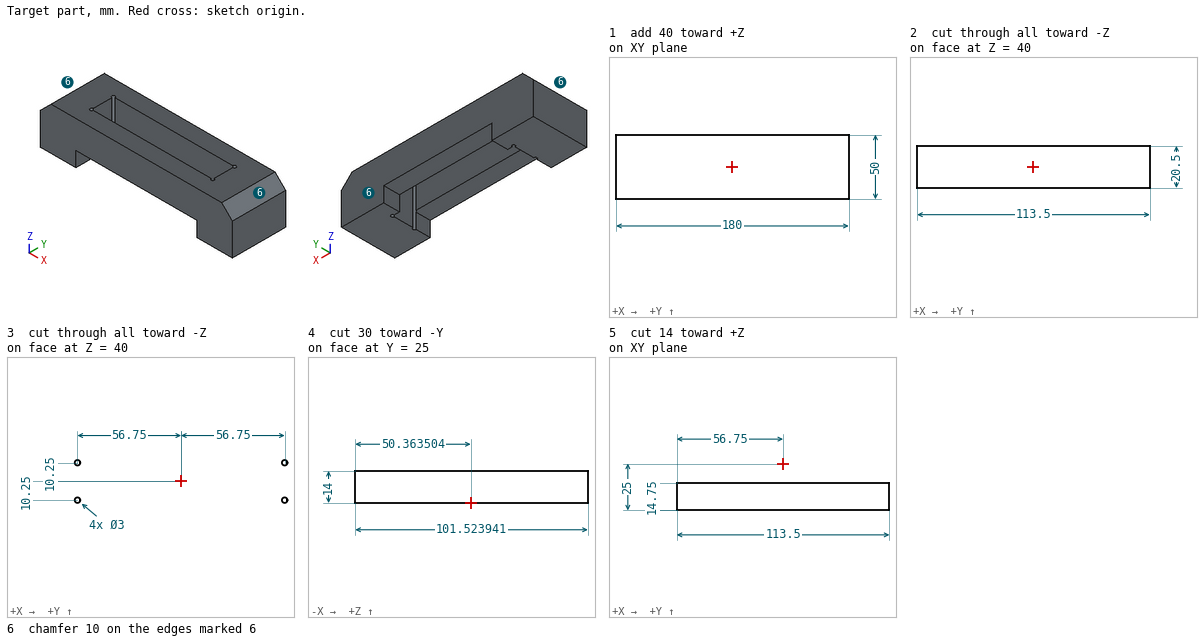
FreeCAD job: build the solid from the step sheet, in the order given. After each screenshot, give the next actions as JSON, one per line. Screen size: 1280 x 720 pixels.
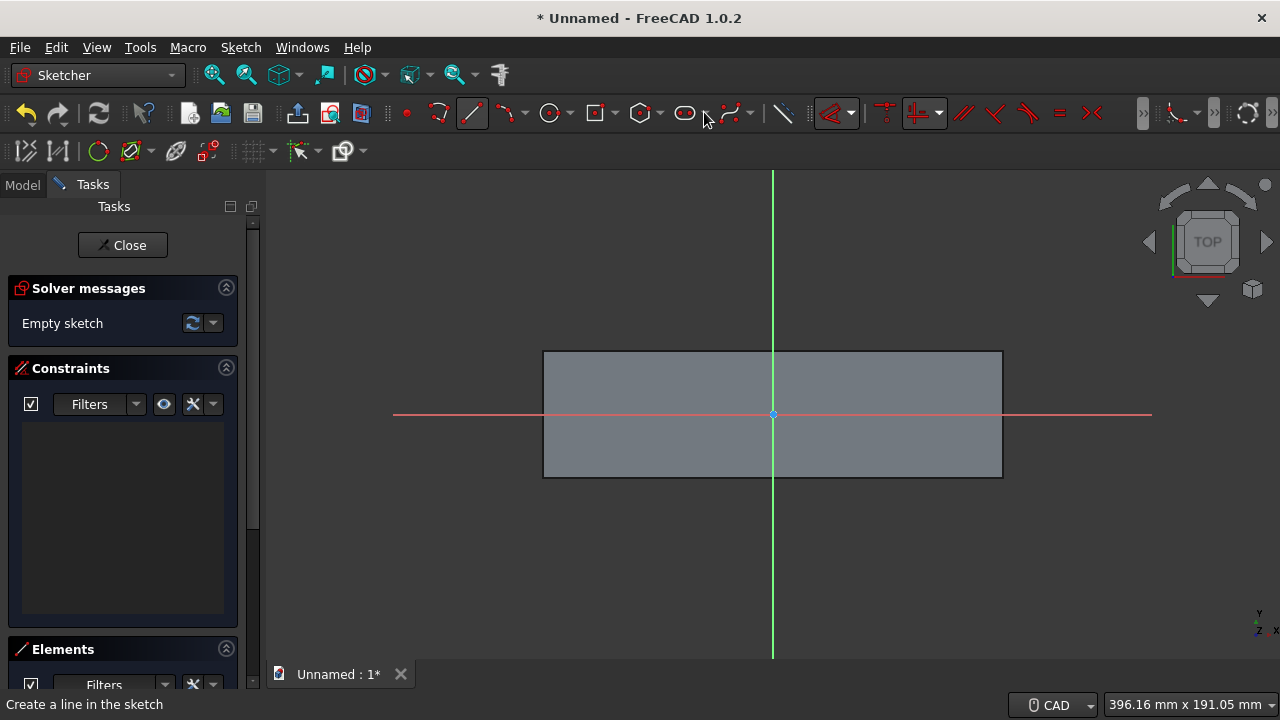
{"action": "scroll", "coordinate": [856, 415], "scroll_direction": "up", "scroll_amount": 3}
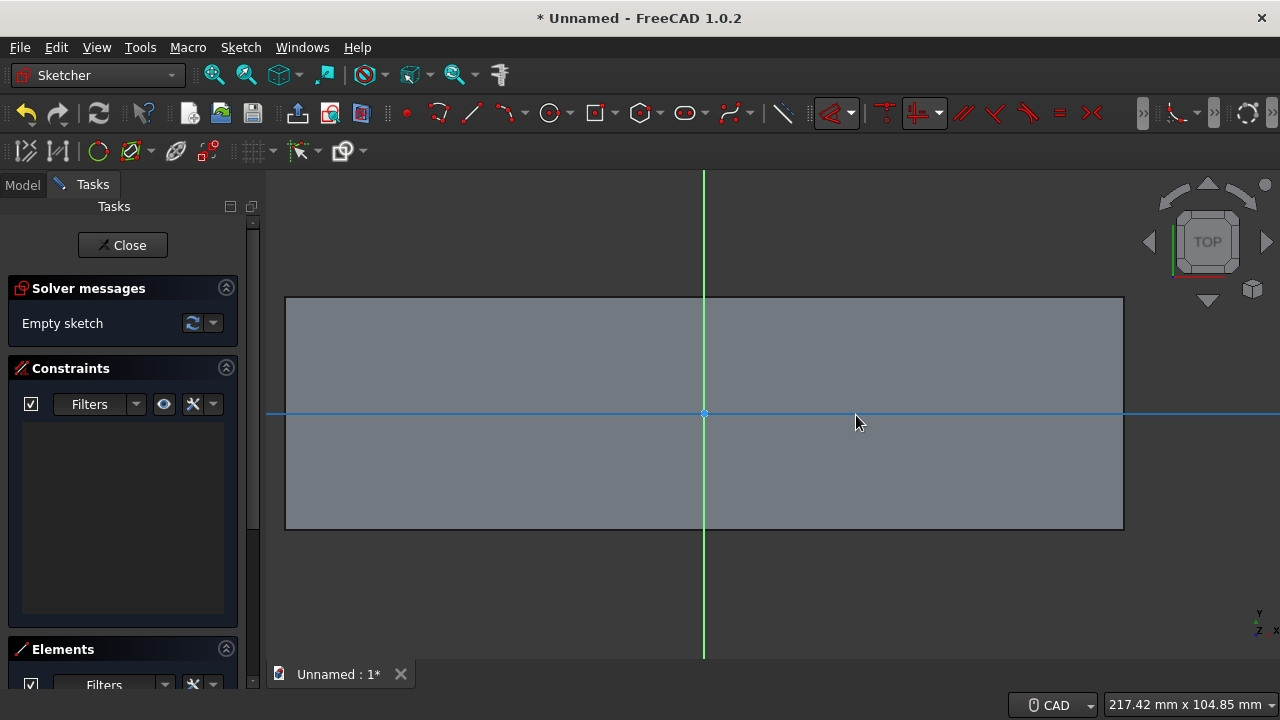
{"action": "key", "text": "g v"}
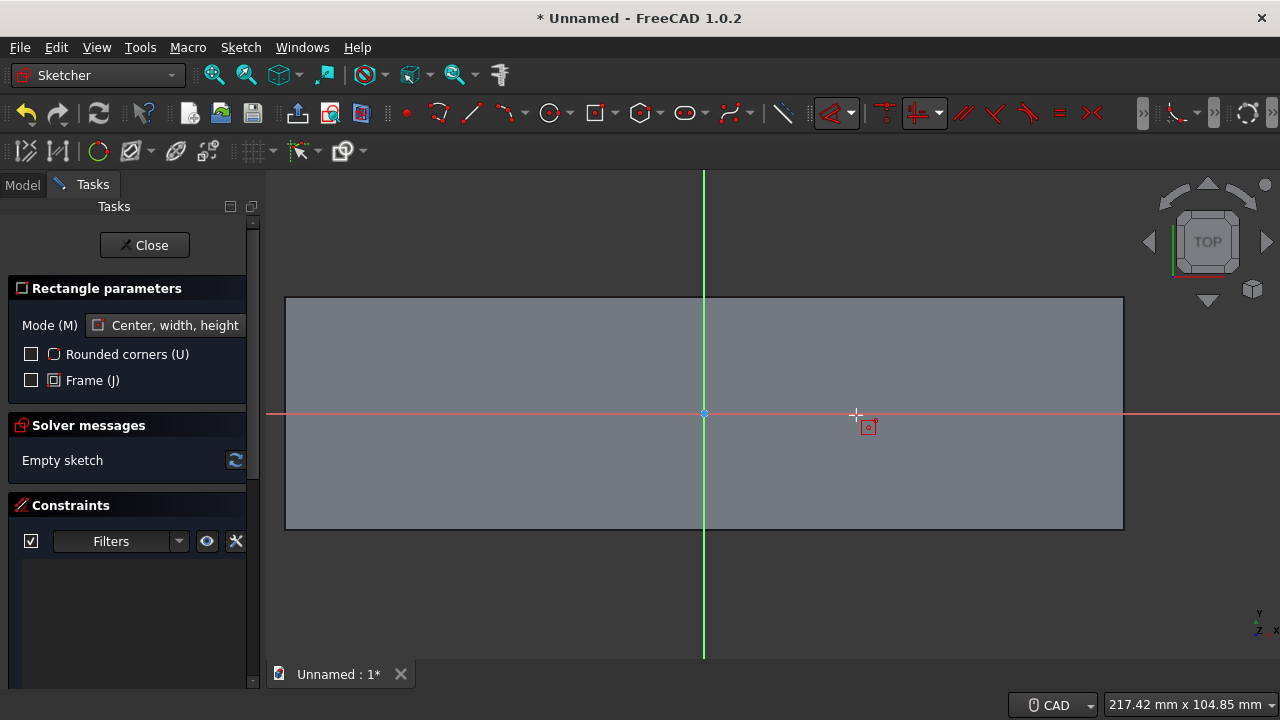
{"action": "left_click", "coordinate": [704, 414]}
{"action": "left_click", "coordinate": [969, 366]}
{"action": "key", "text": "Escape"}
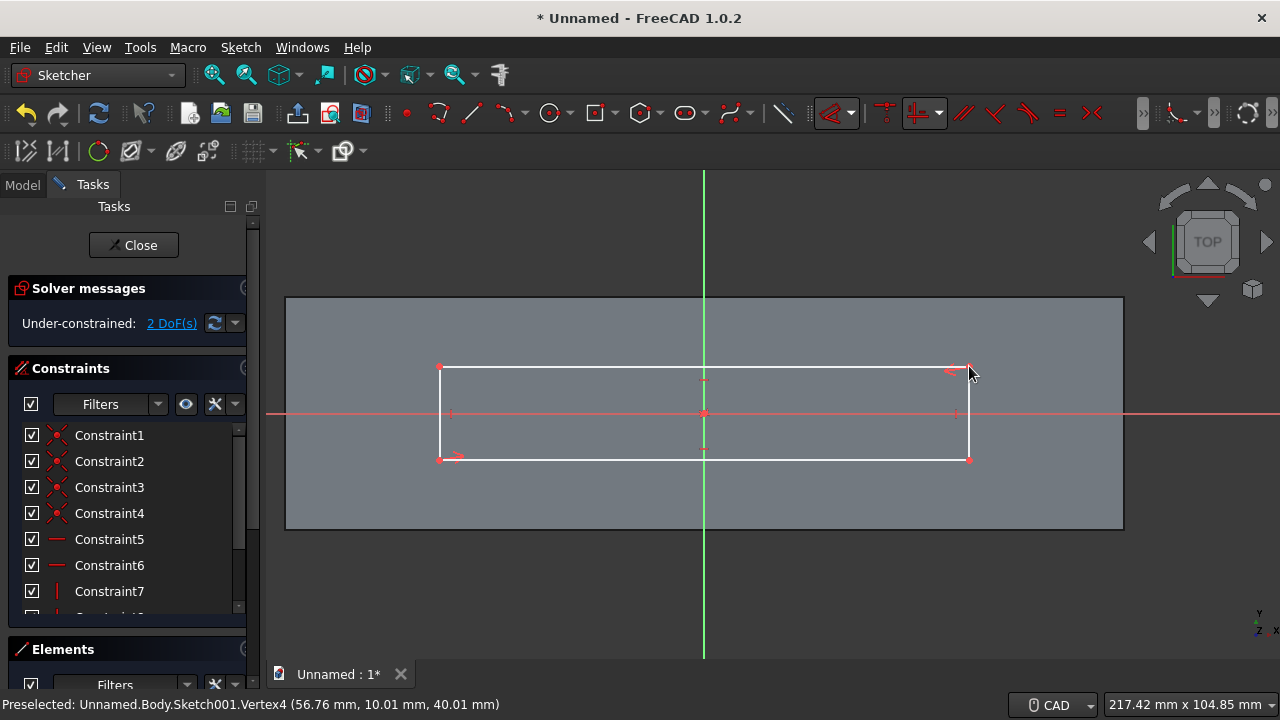
{"action": "left_click", "coordinate": [969, 432]}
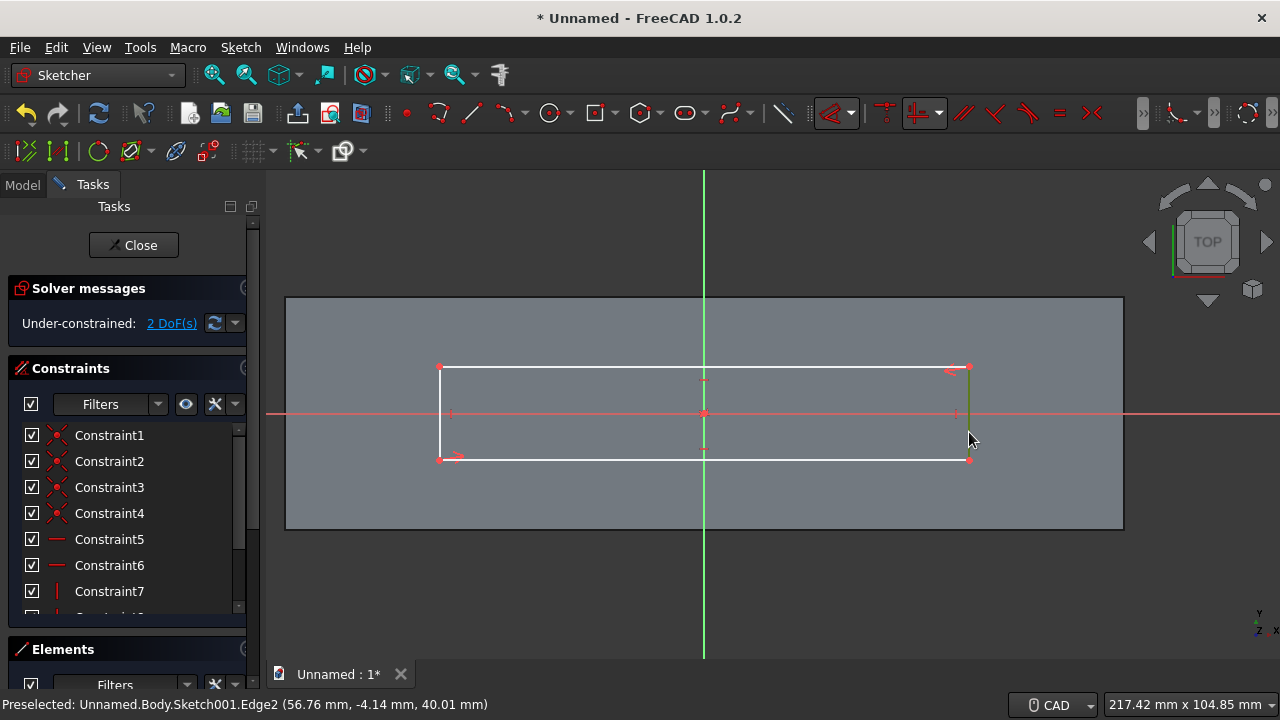
{"action": "key", "text": "i"}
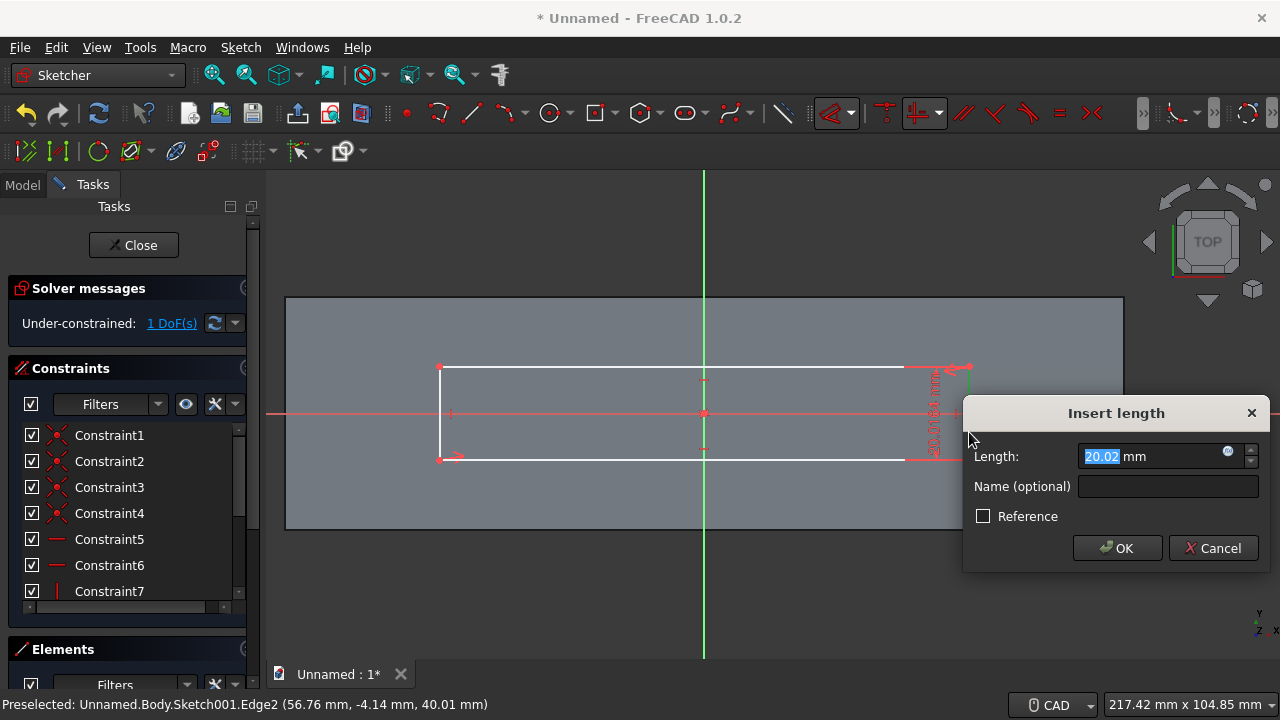
{"action": "type", "text": "20.5"}
{"action": "key", "text": "Return"}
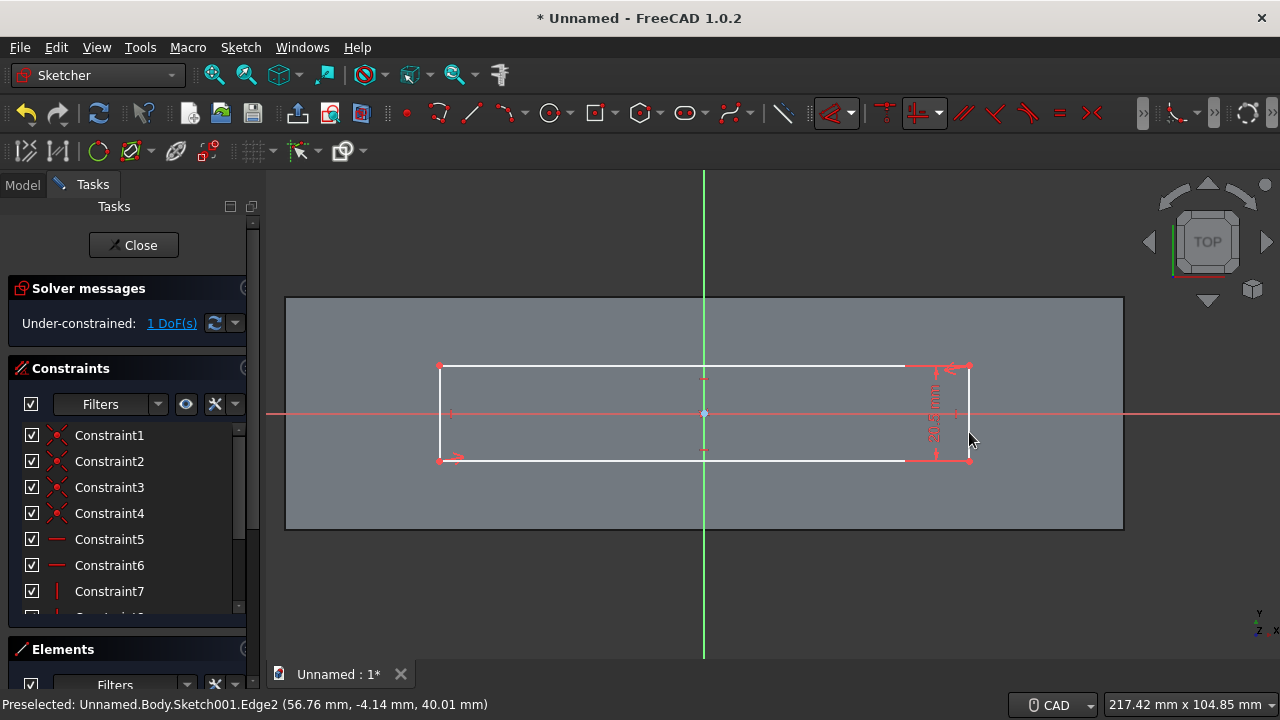
{"action": "left_click", "coordinate": [598, 461]}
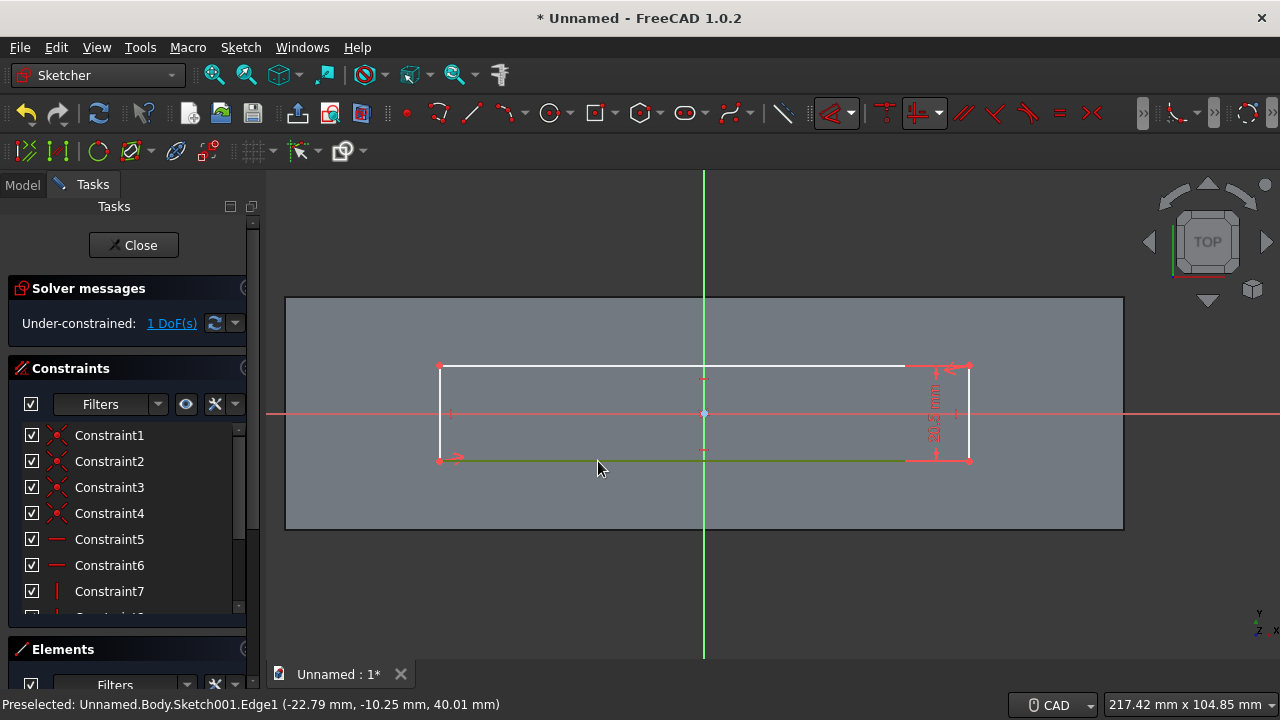
{"action": "left_click", "coordinate": [854, 114]}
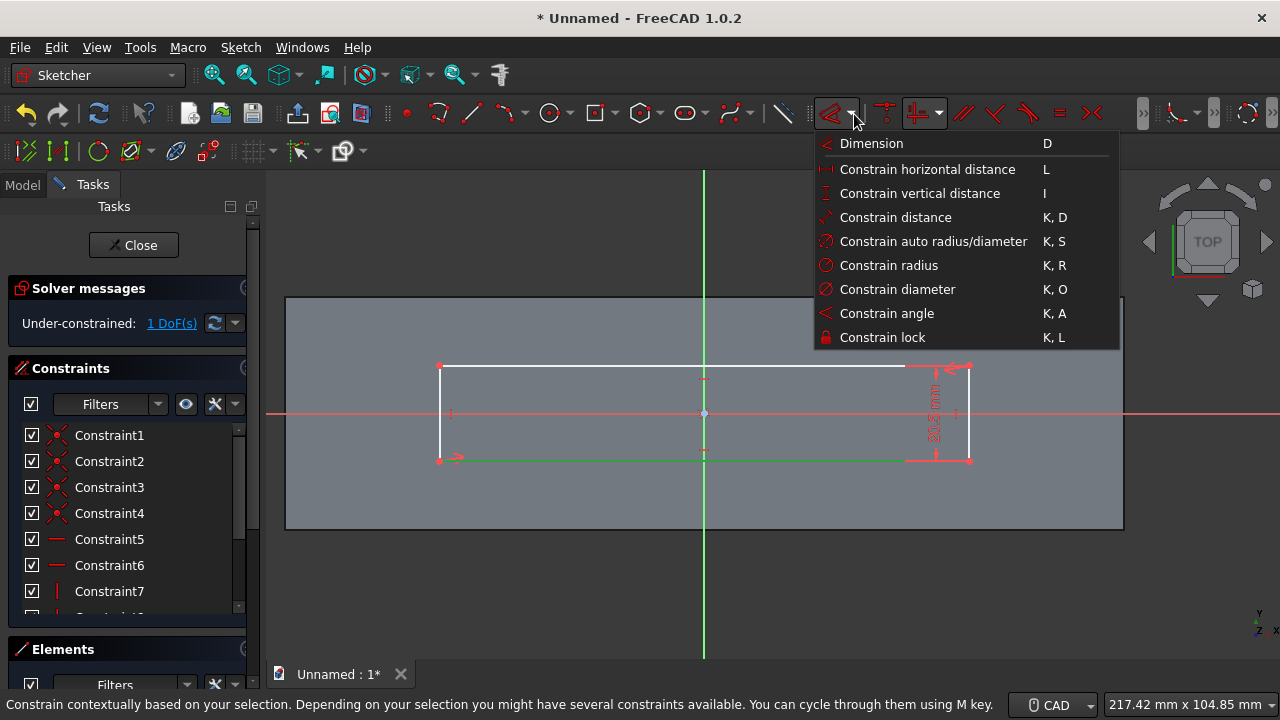
{"action": "left_click", "coordinate": [967, 169]}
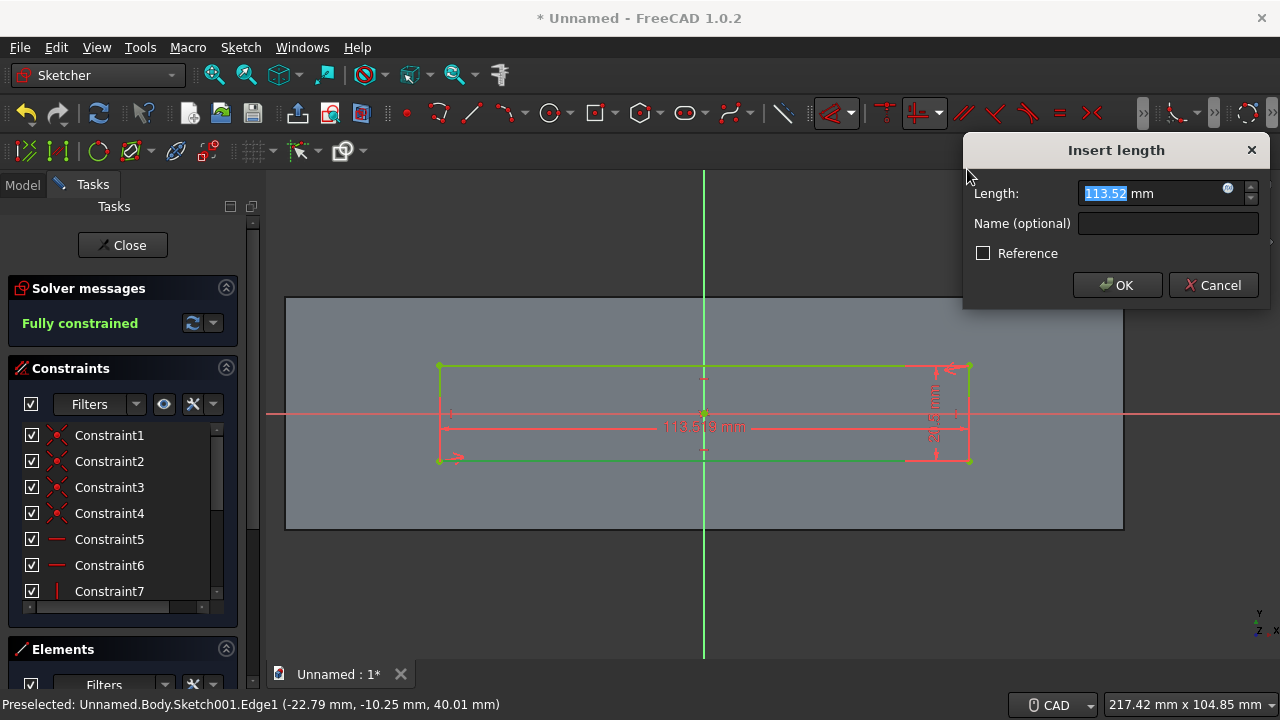
{"action": "type", "text": "113.5"}
{"action": "key", "text": "Return"}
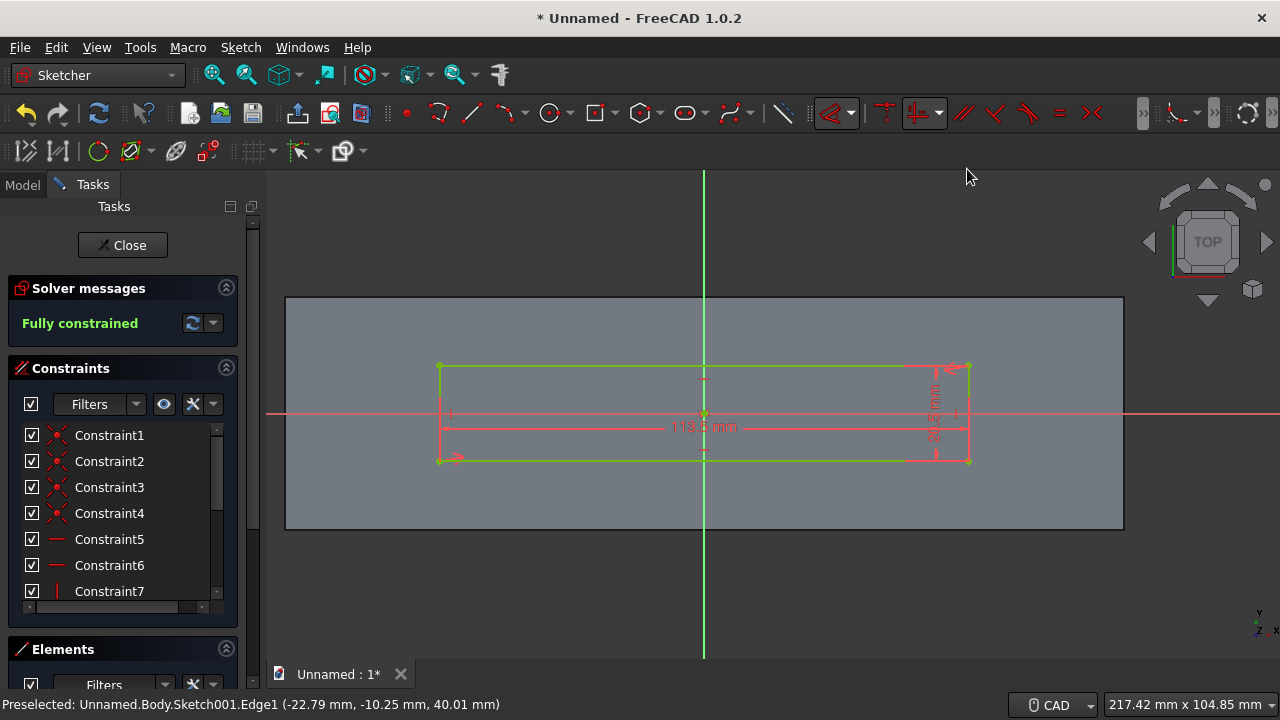
{"action": "left_click", "coordinate": [123, 245]}